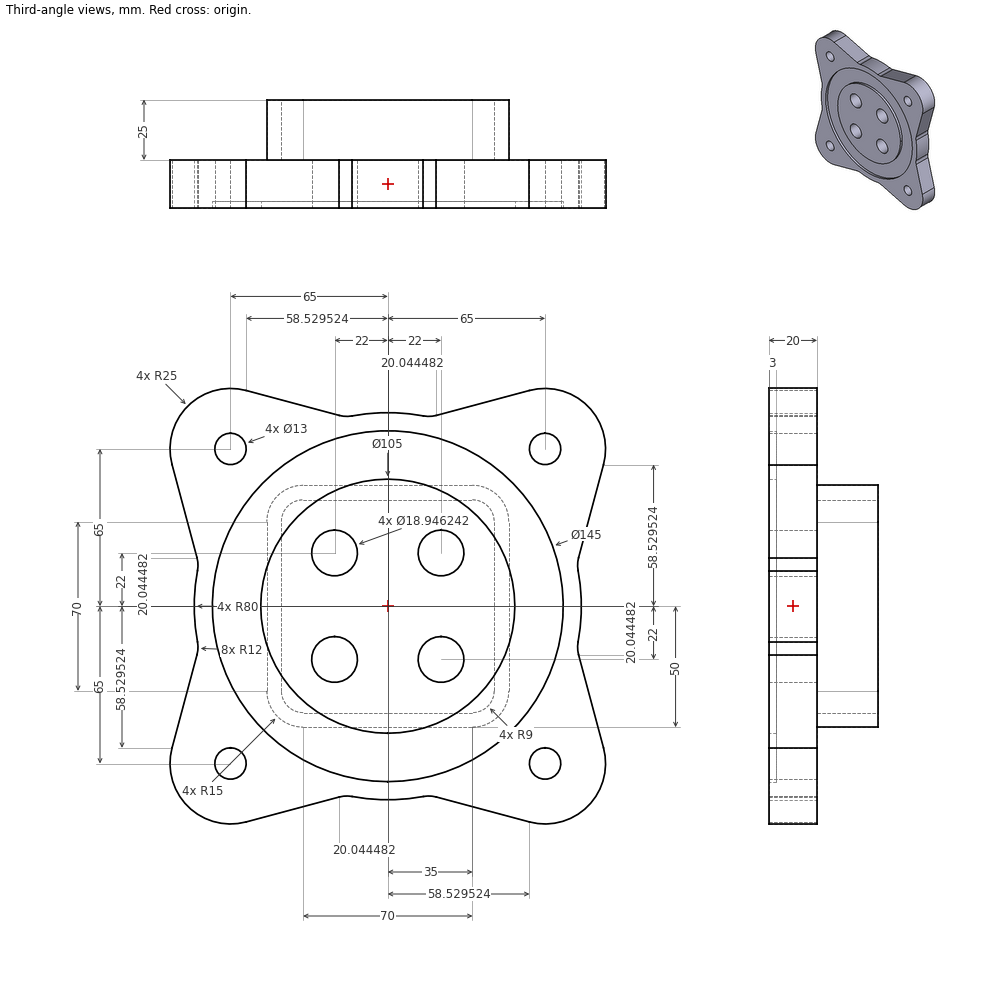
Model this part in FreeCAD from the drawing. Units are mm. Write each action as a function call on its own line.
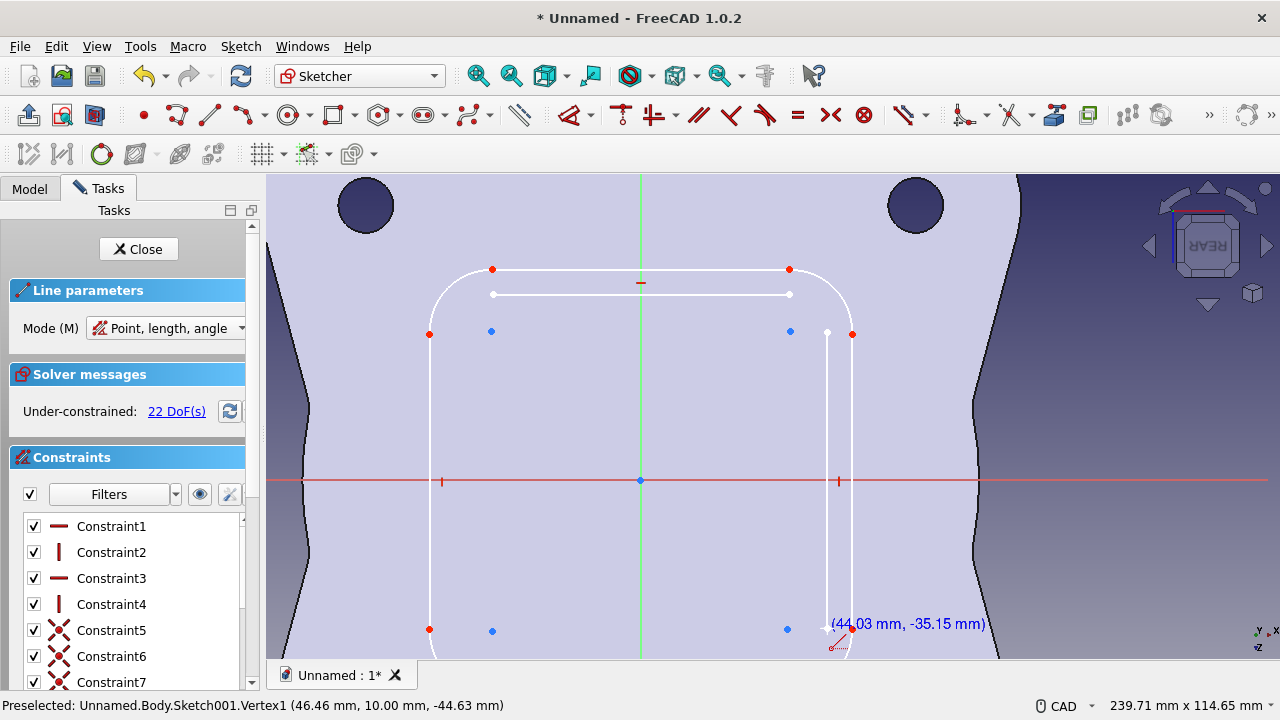
scroll(834, 287, down, 2)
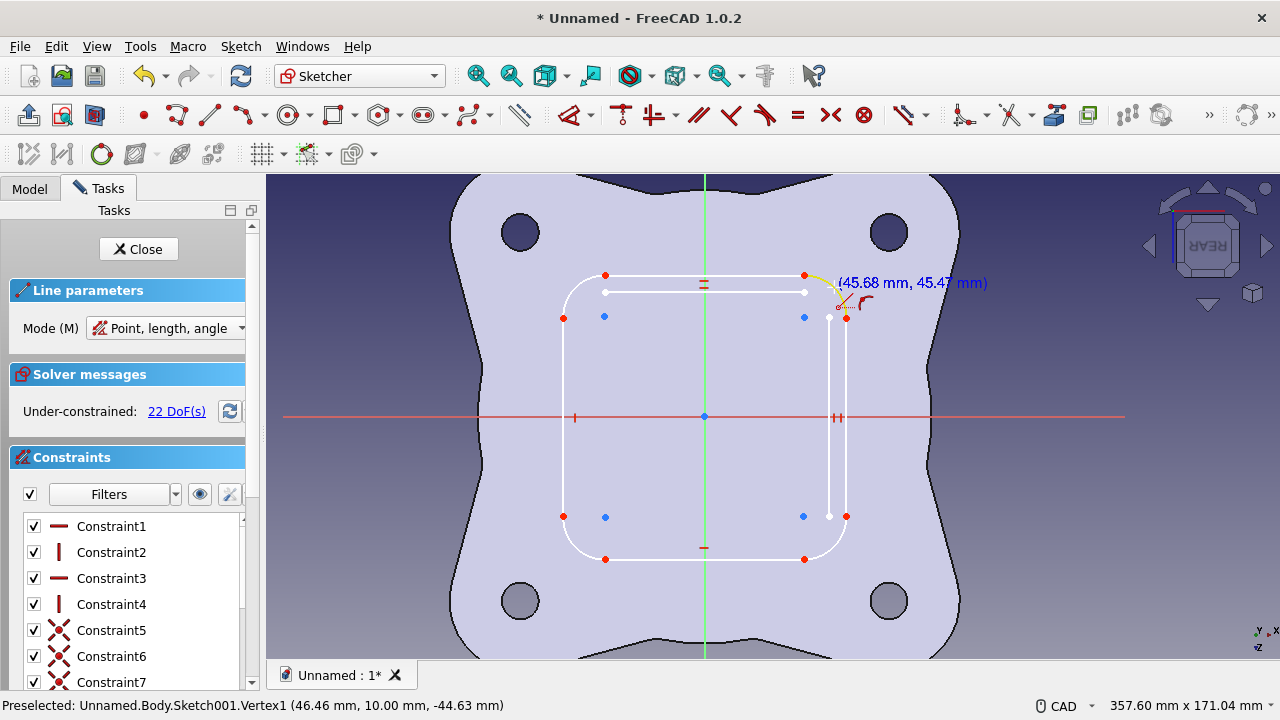
click(804, 541)
click(605, 541)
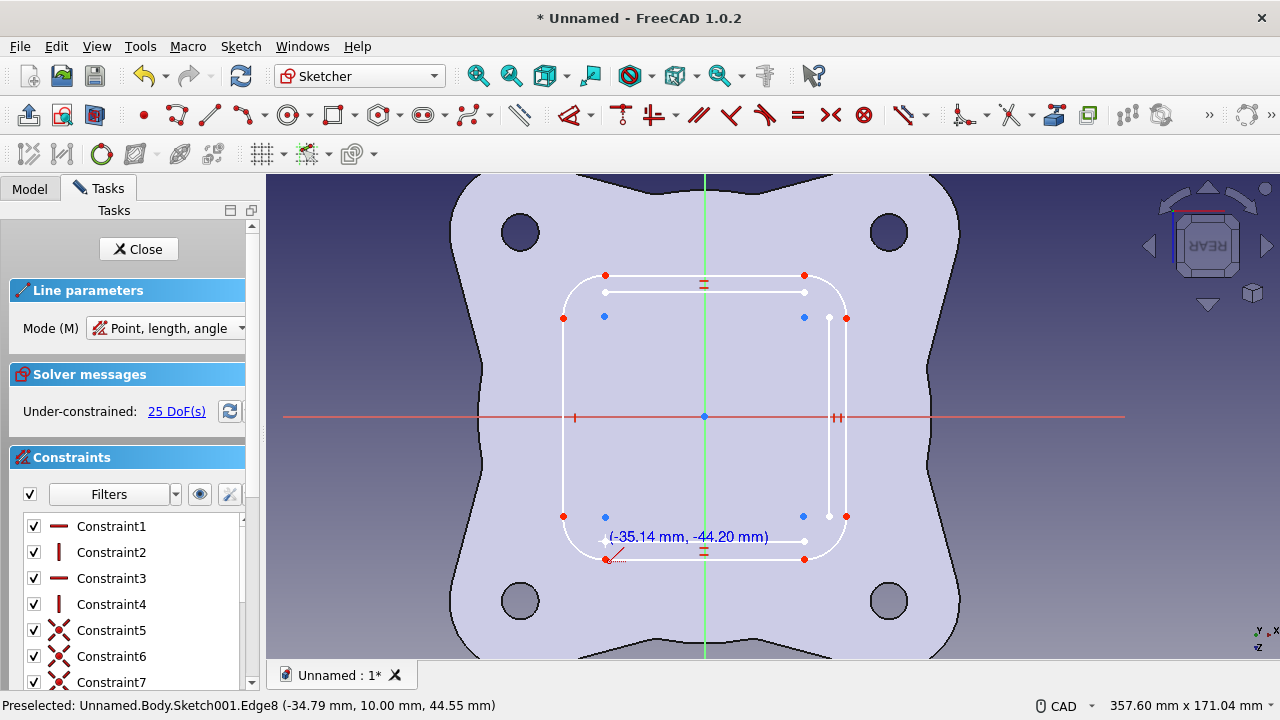
click(580, 516)
click(580, 317)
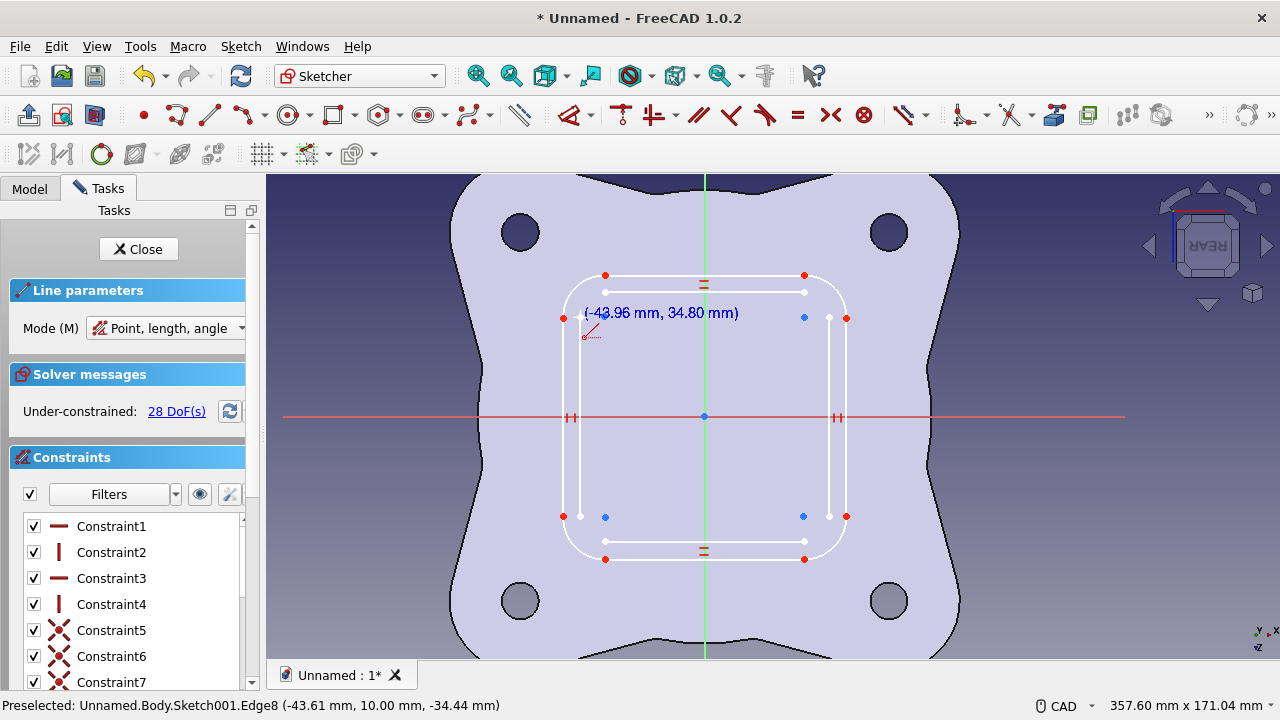
click(242, 116)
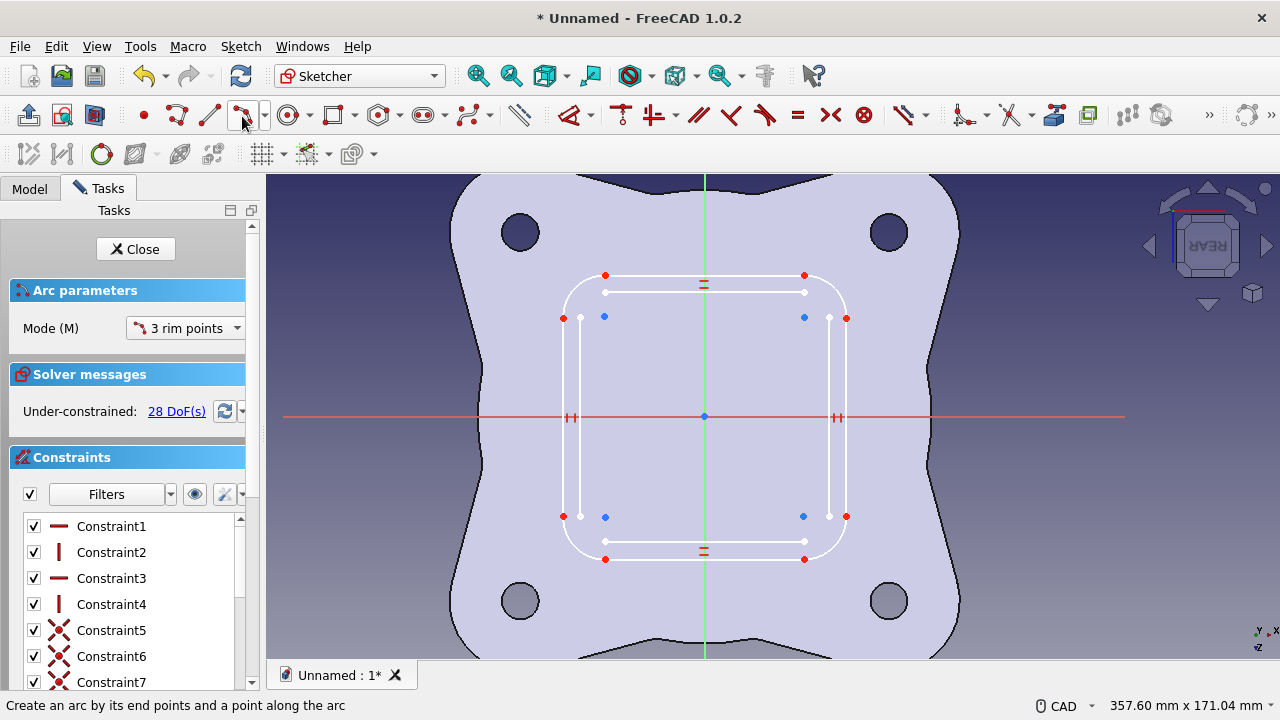
click(804, 292)
click(829, 318)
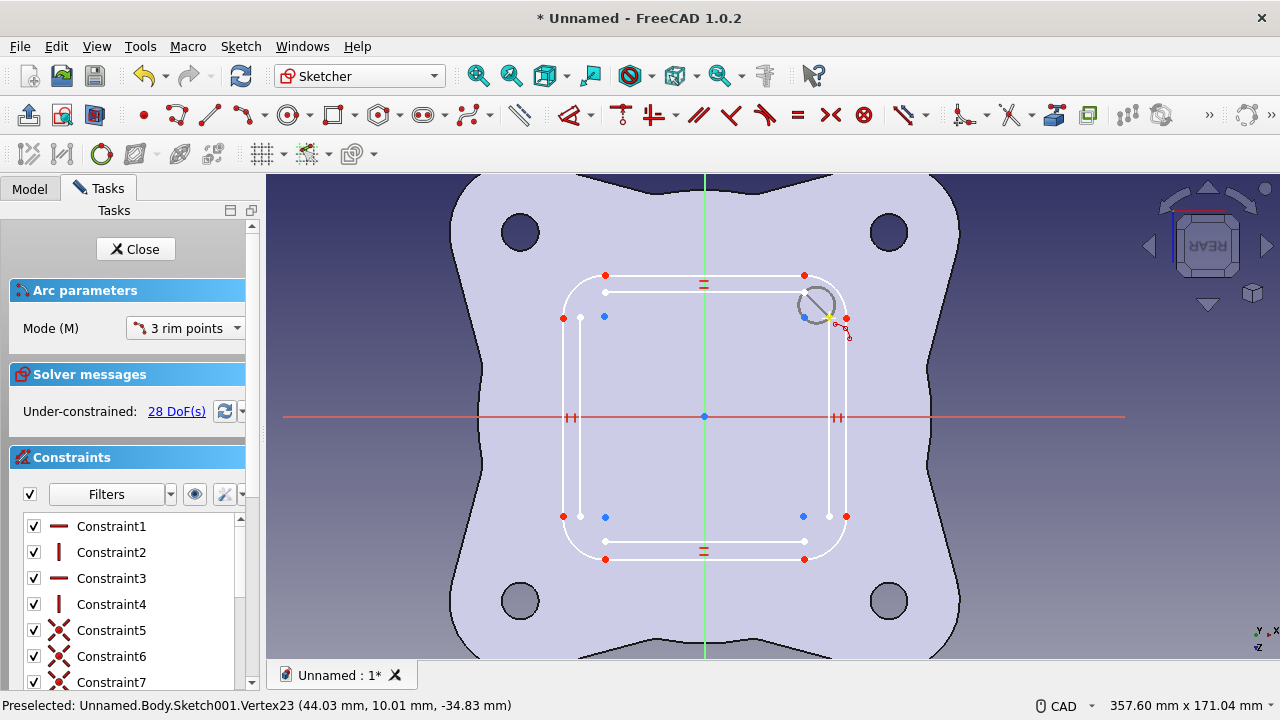
scroll(822, 299, up, 4)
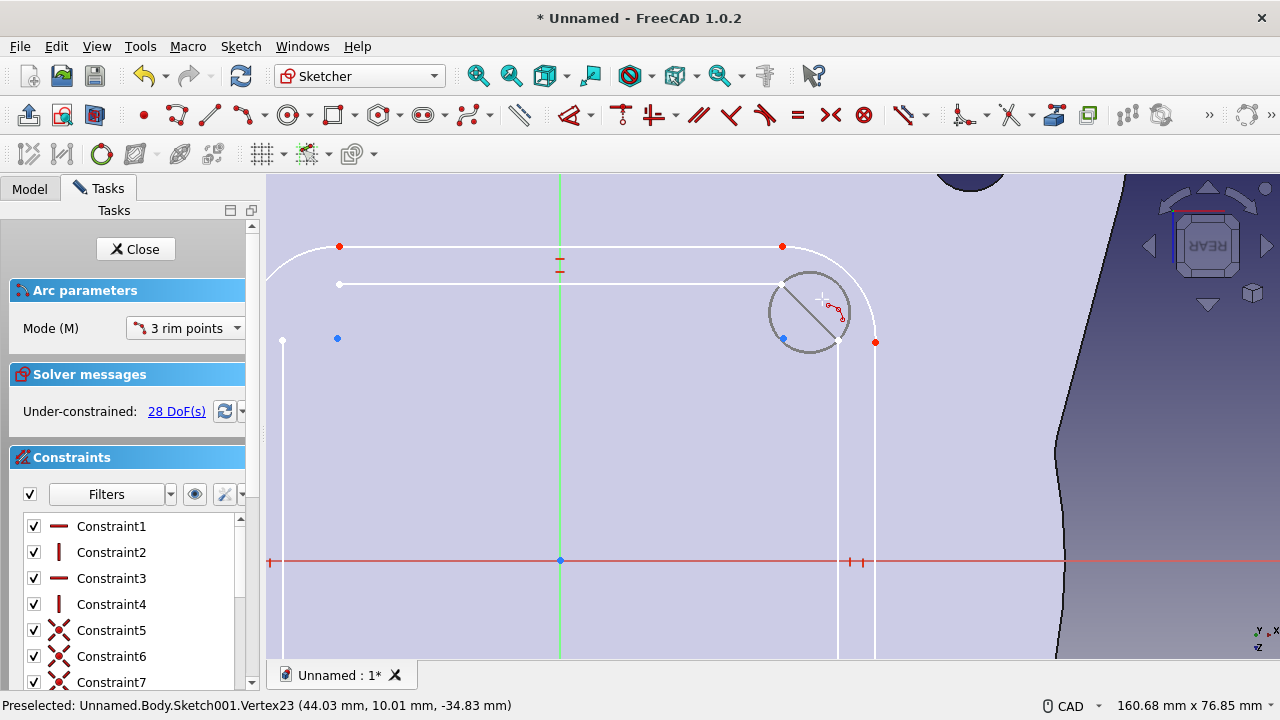
click(821, 300)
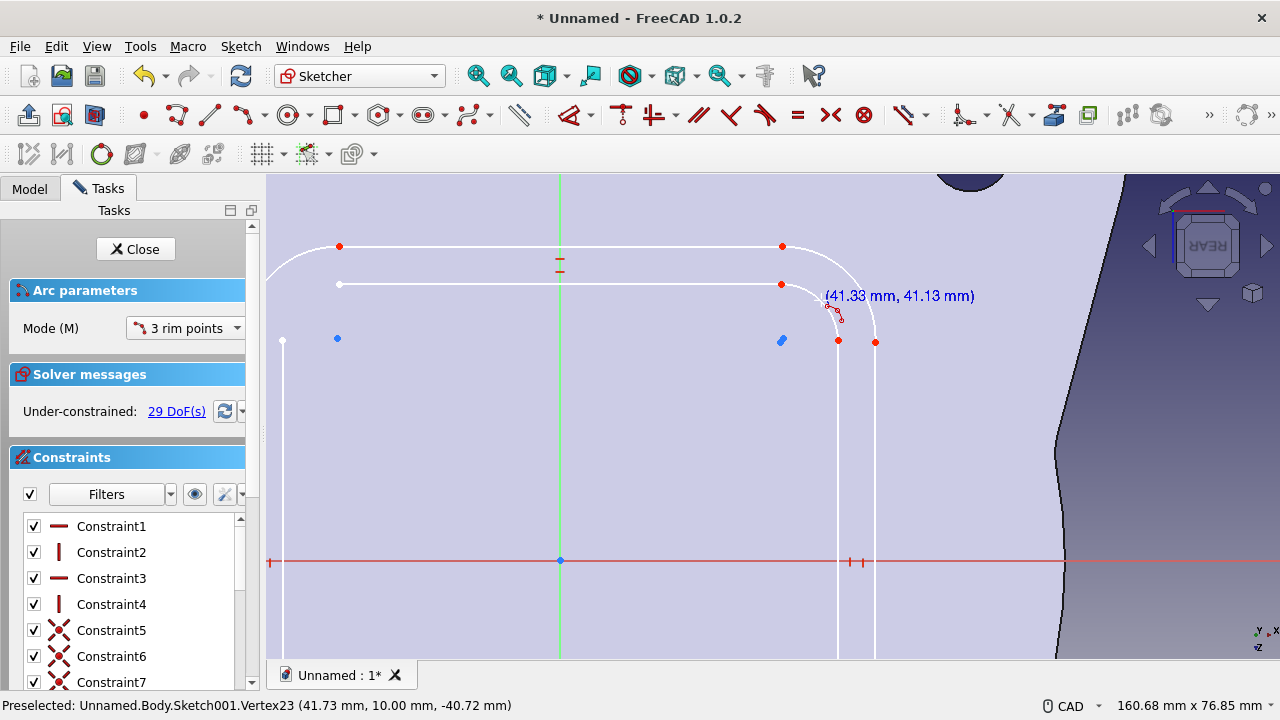
scroll(822, 299, down, 4)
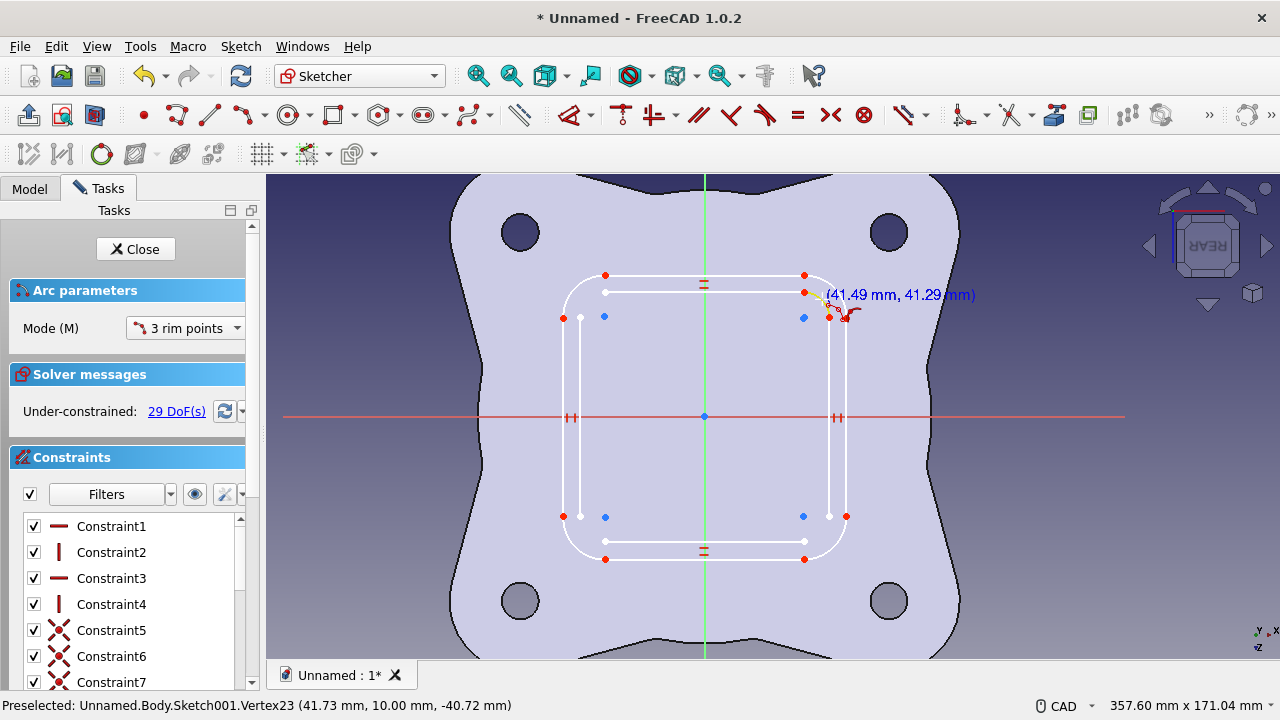
click(829, 516)
click(804, 542)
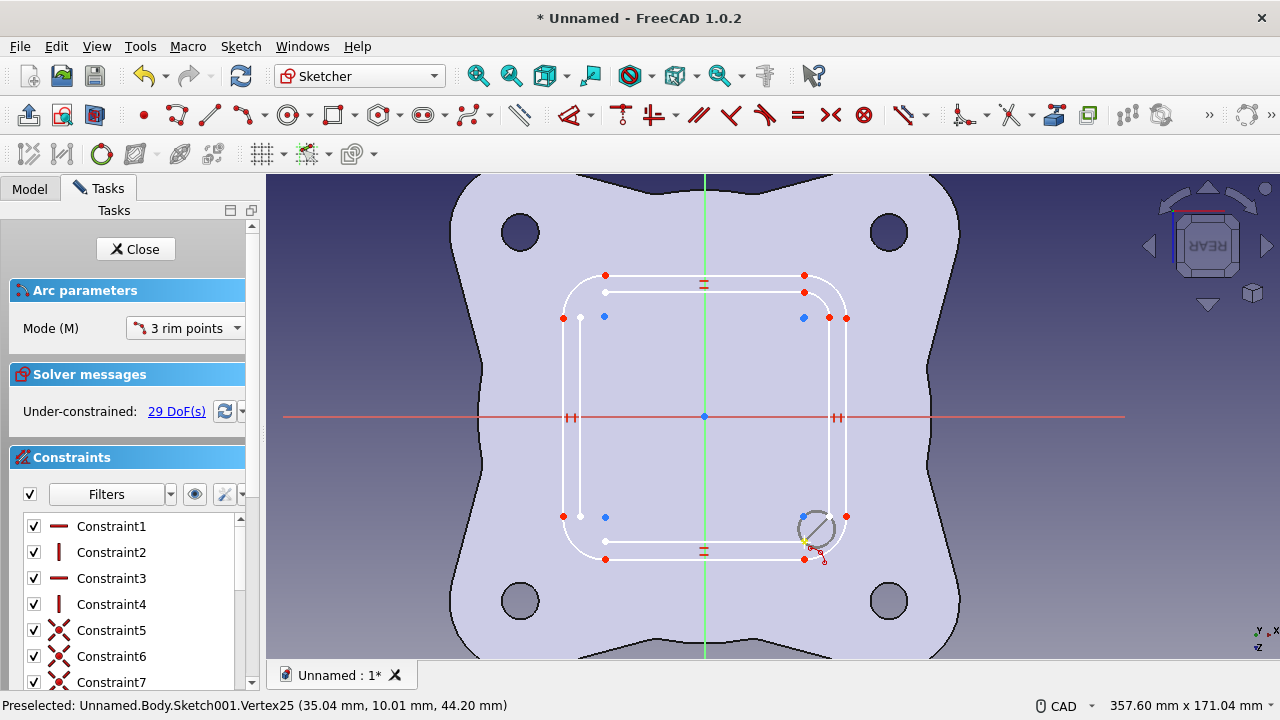
scroll(822, 534, up, 4)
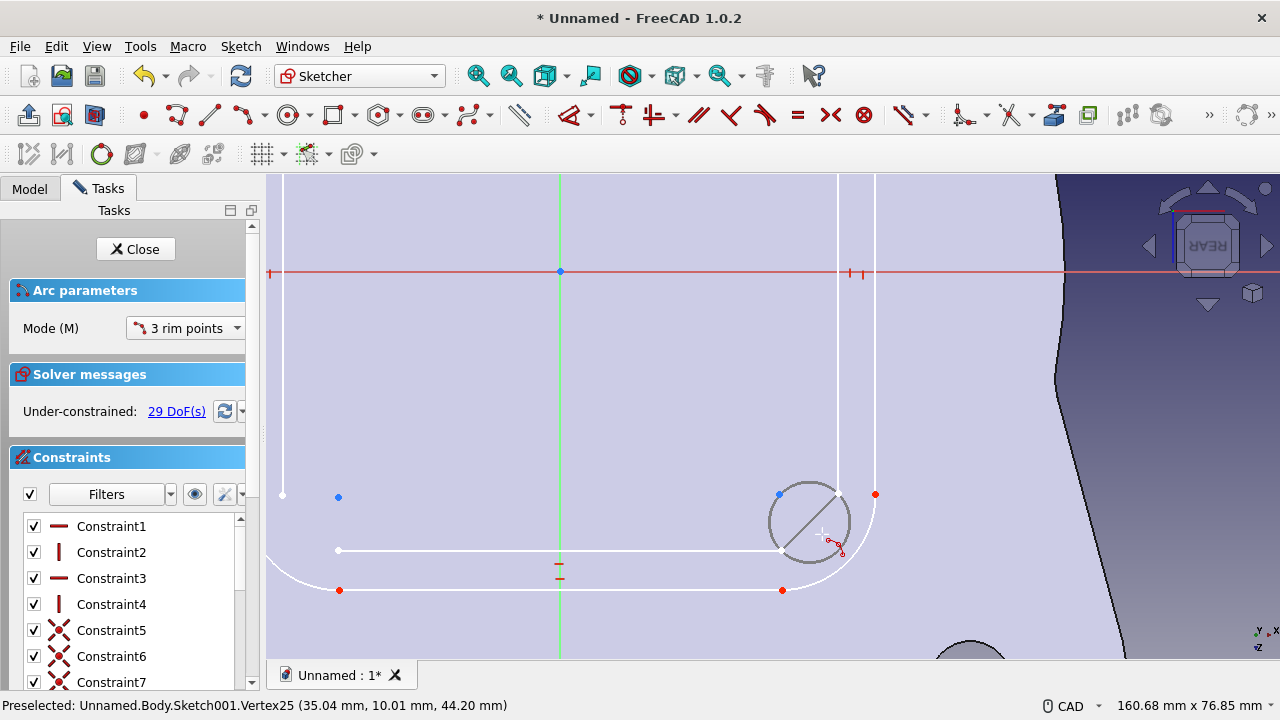
click(821, 533)